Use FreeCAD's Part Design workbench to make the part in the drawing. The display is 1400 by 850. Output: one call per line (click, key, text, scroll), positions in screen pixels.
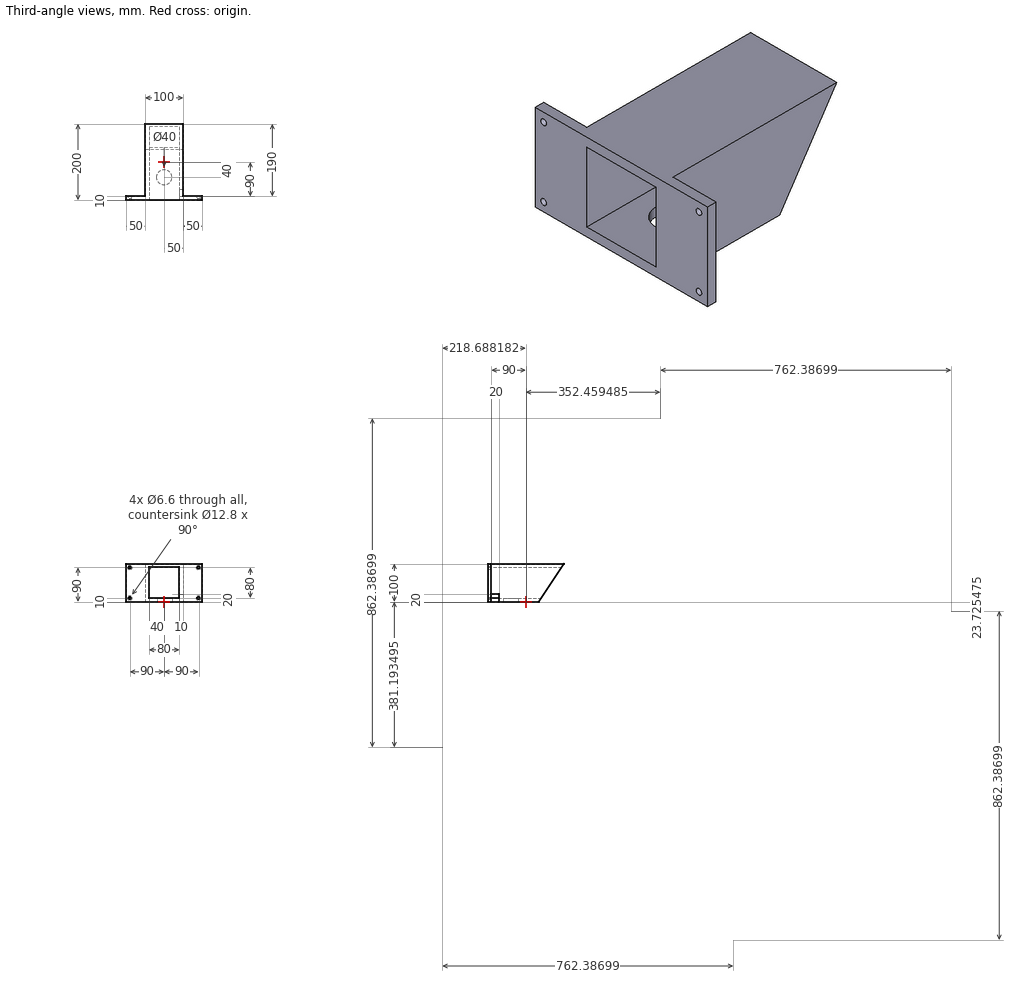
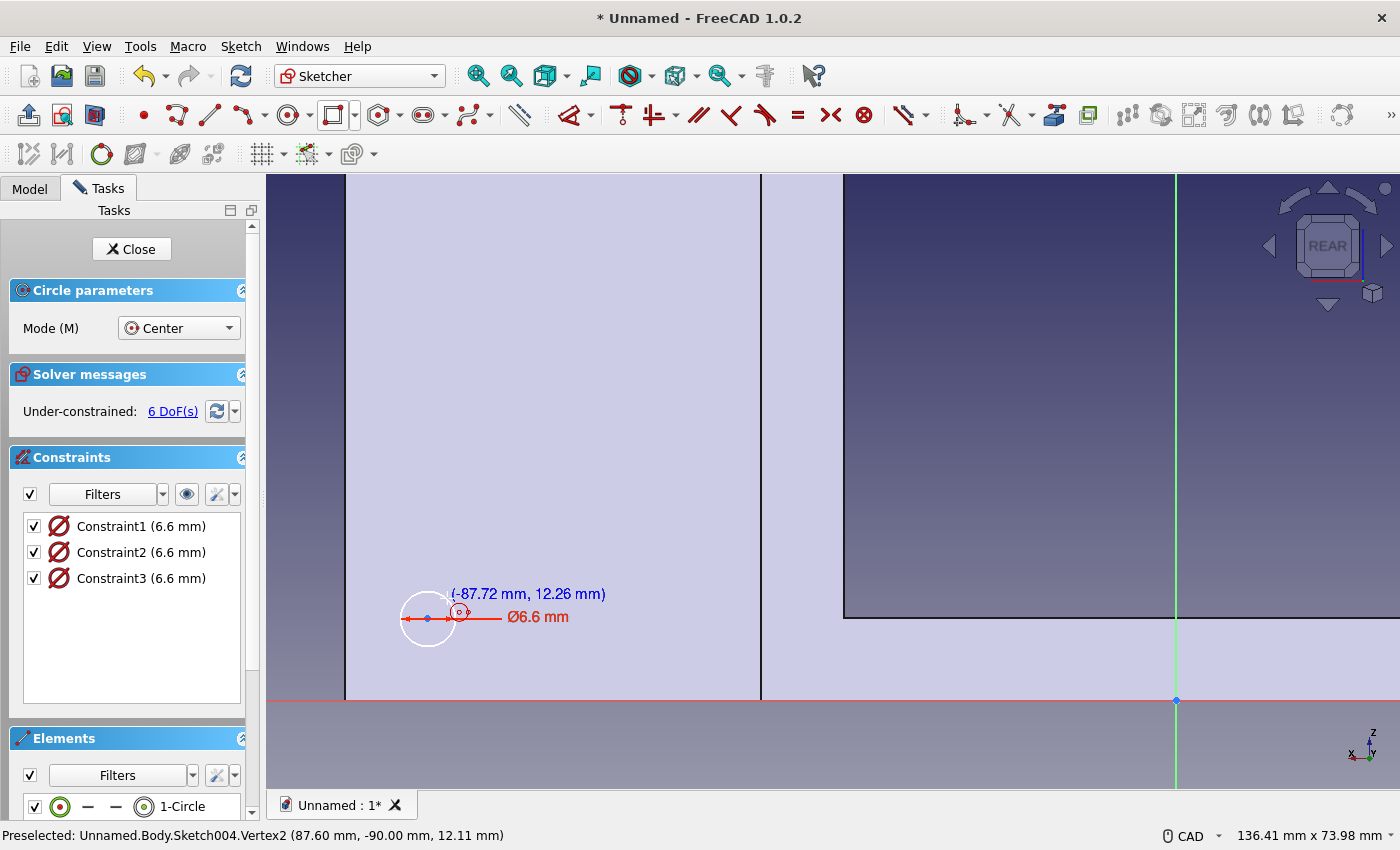
scroll(429, 619, down, 4)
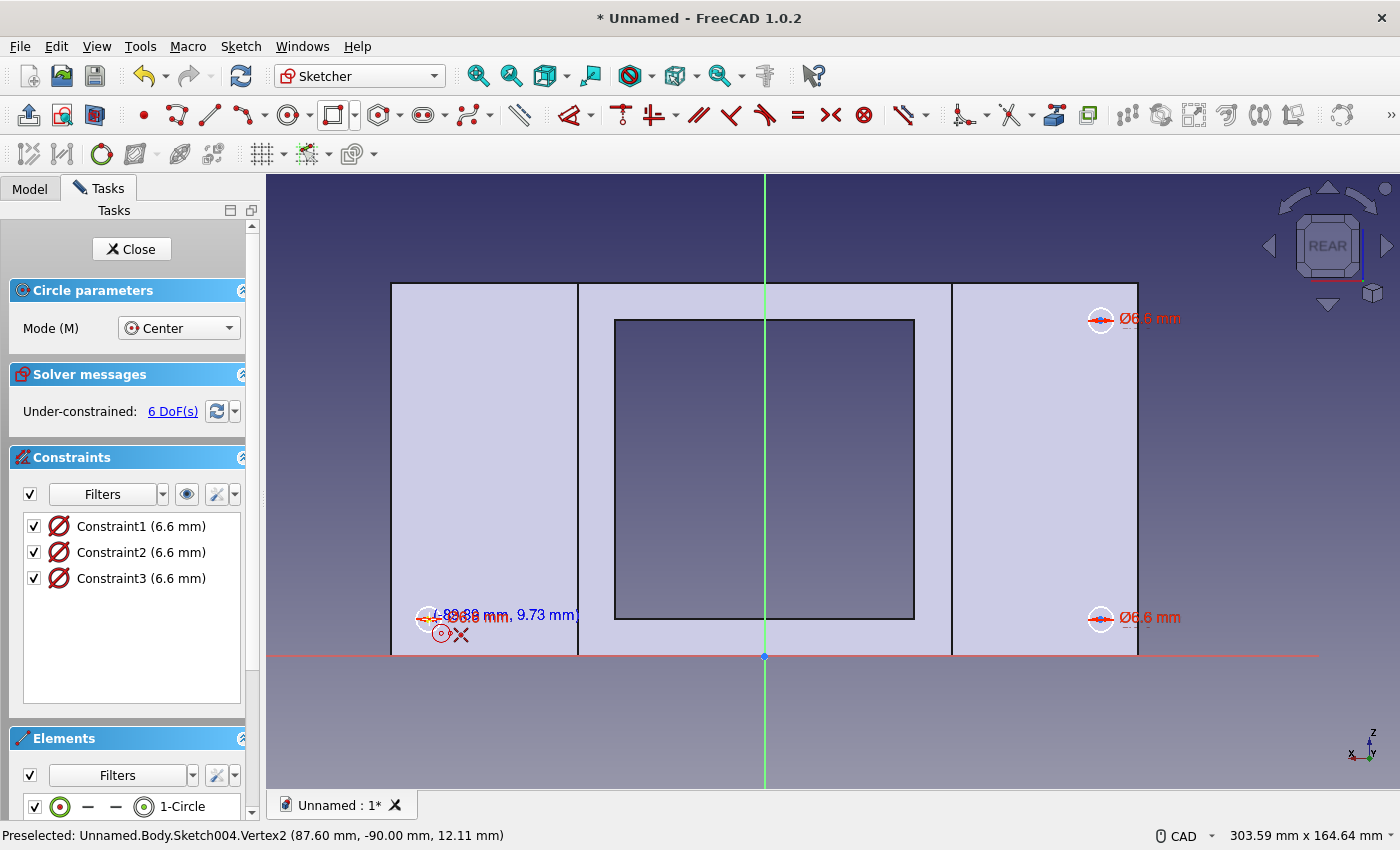
scroll(429, 320, up, 4)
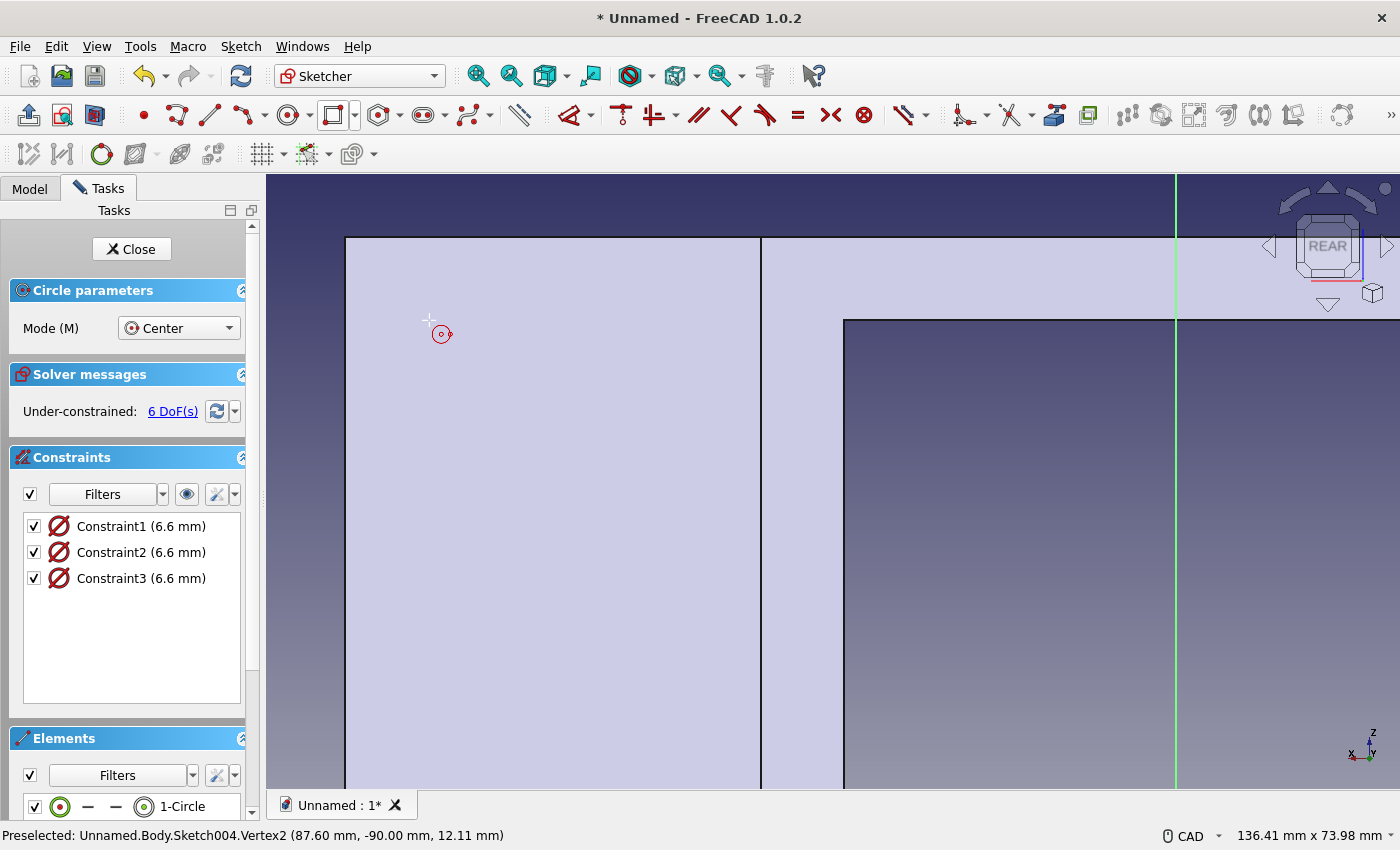
click(428, 320)
move(447, 300)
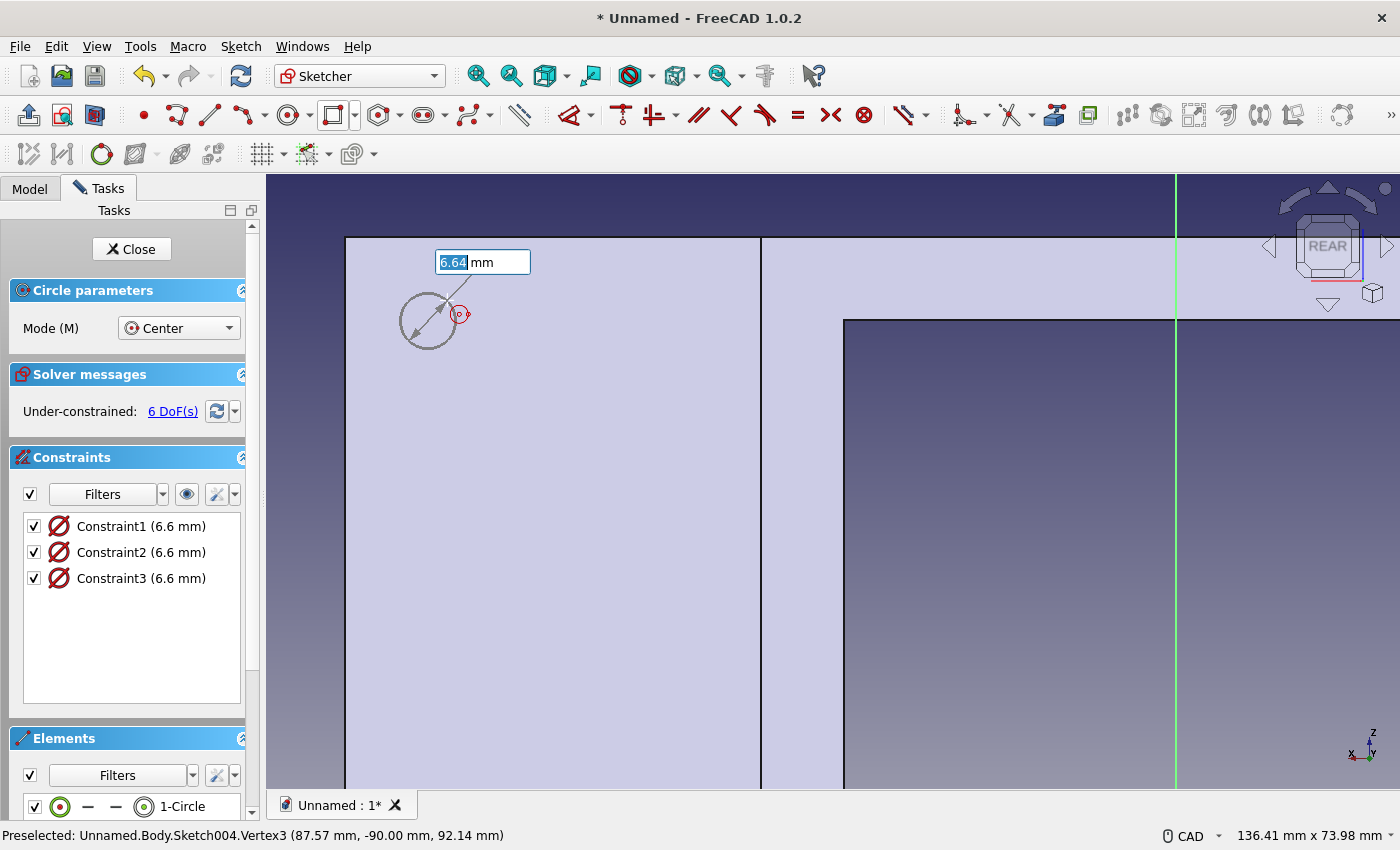
text(6.6)
key(Return)
key(Escape)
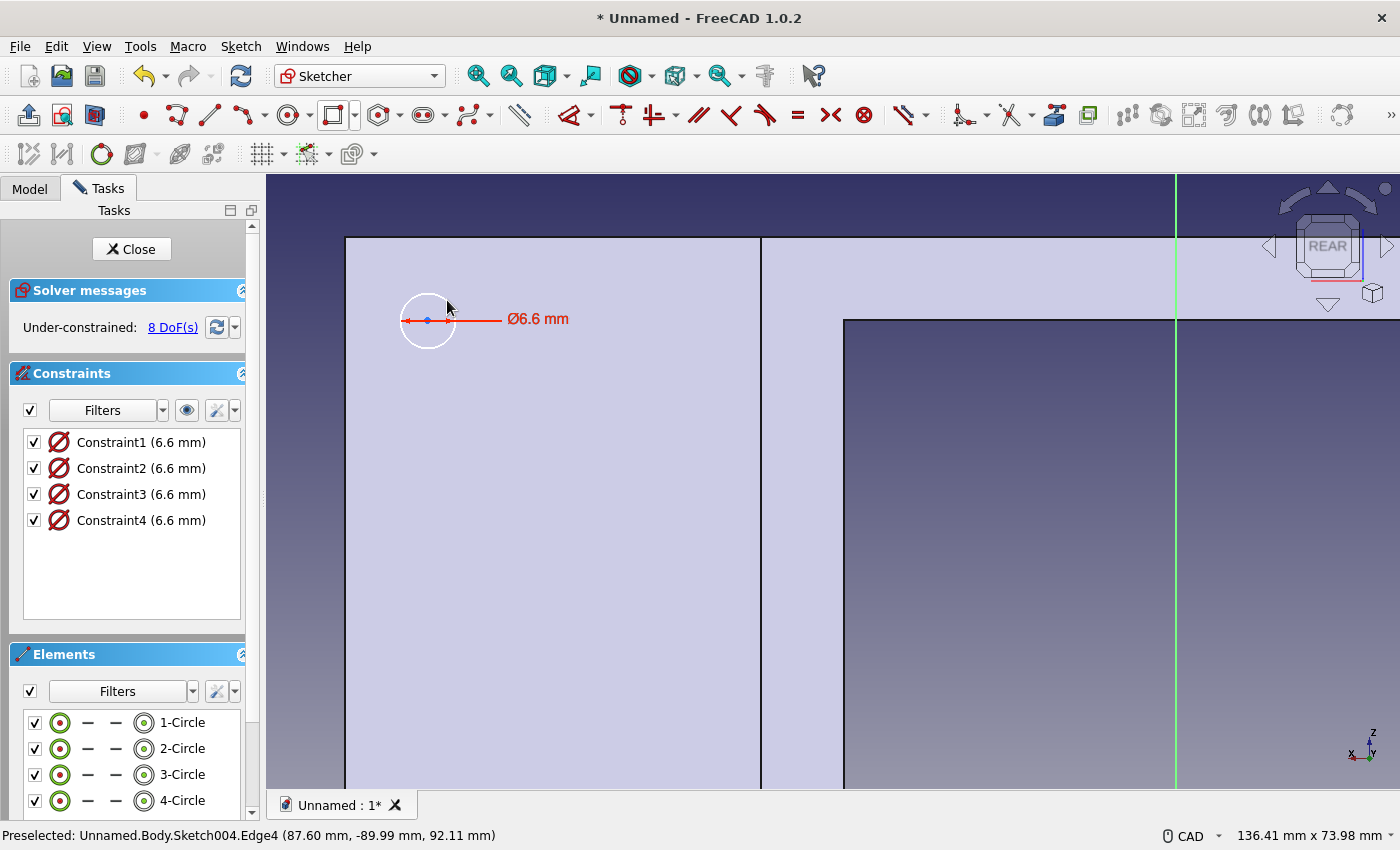
scroll(429, 319, down, 4)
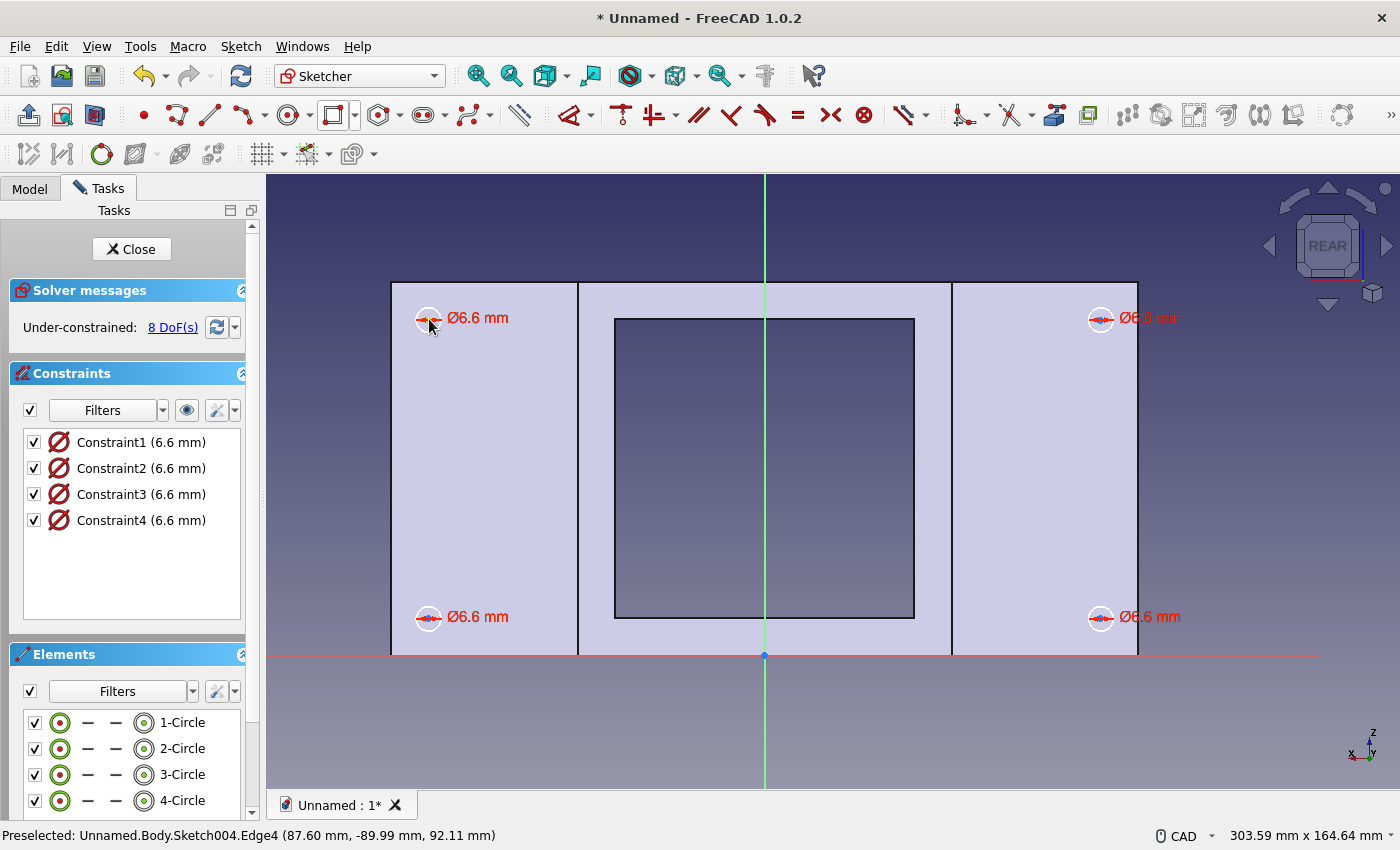
click(1101, 619)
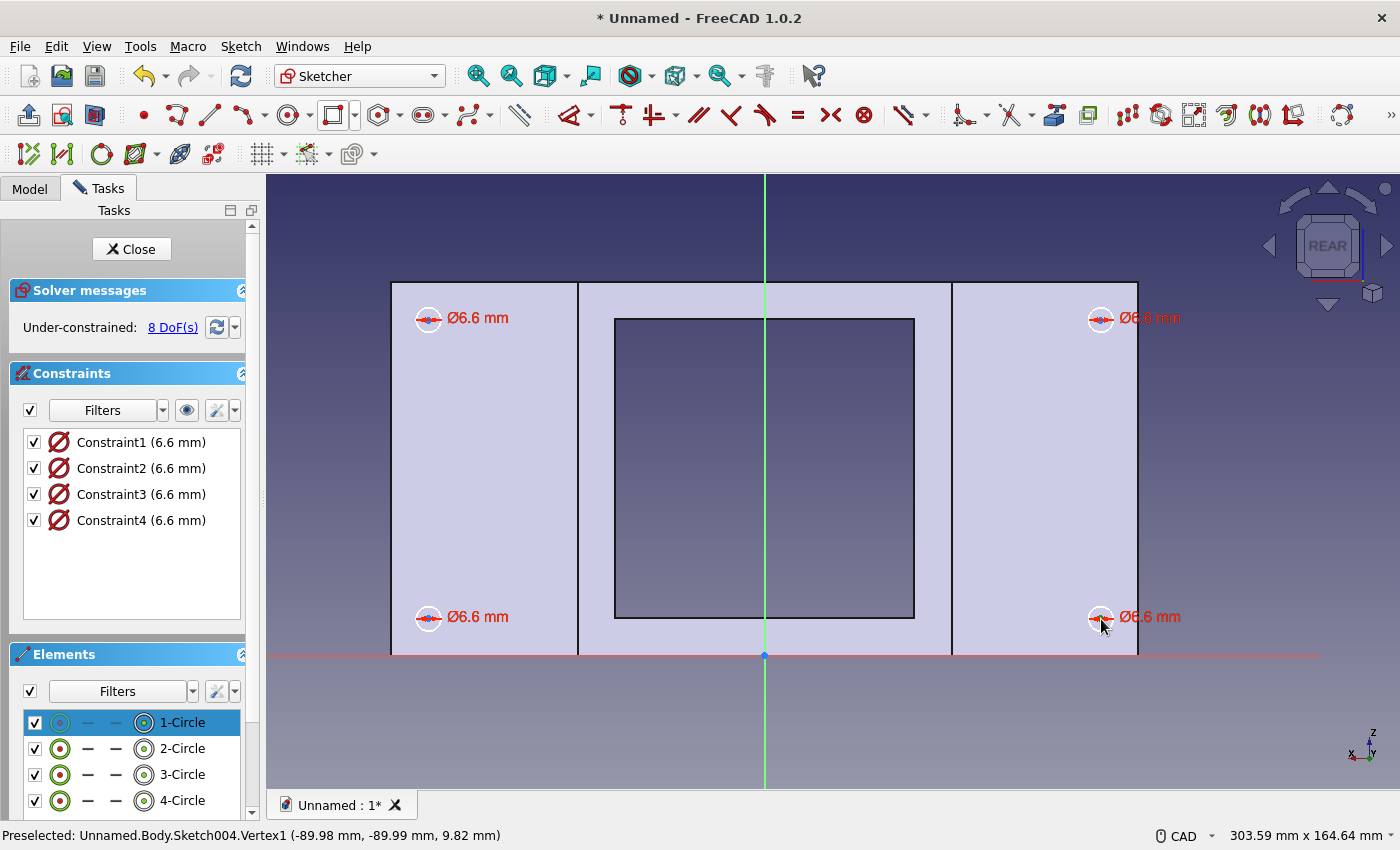
click(1101, 320)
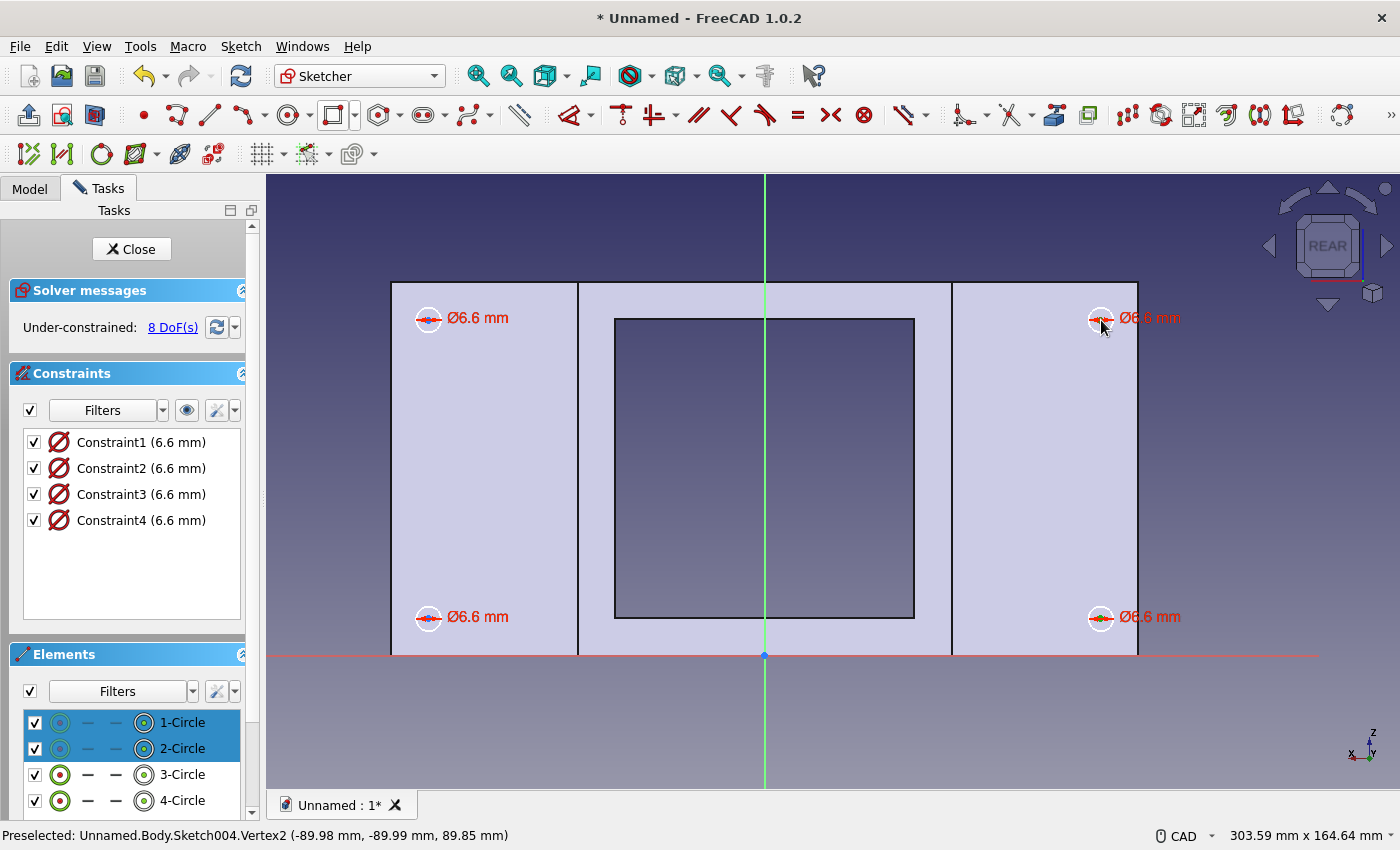
key(v)